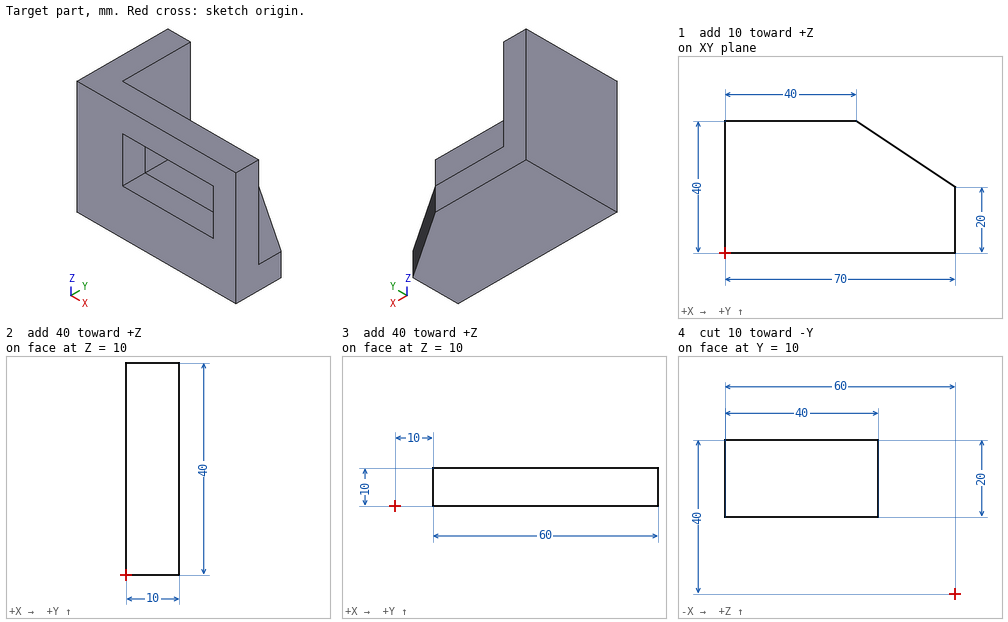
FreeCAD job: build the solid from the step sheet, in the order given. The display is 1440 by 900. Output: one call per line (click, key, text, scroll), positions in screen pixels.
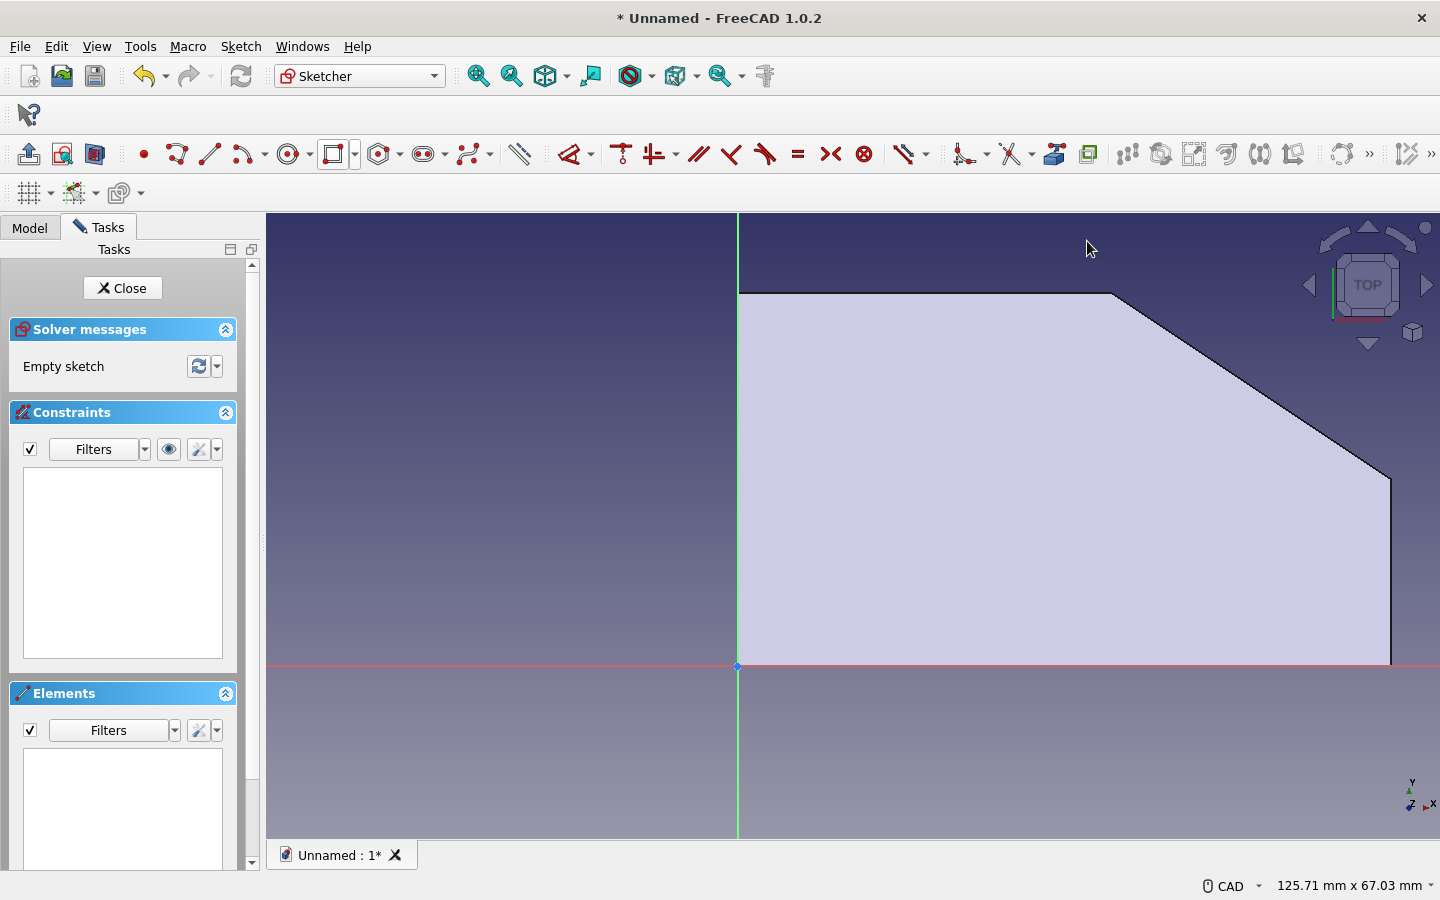
click(332, 154)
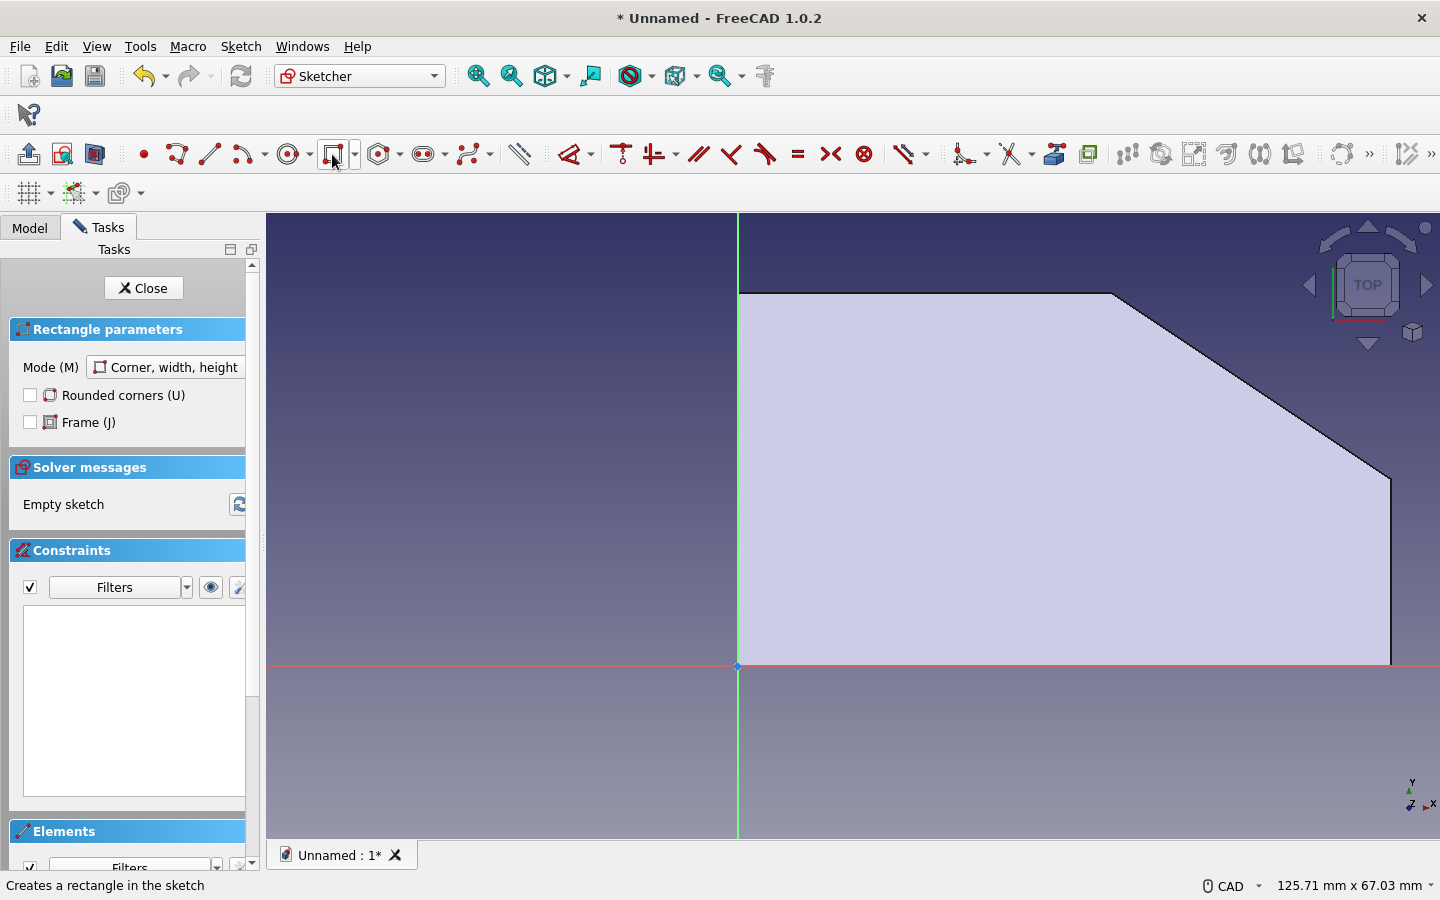
click(738, 666)
move(831, 293)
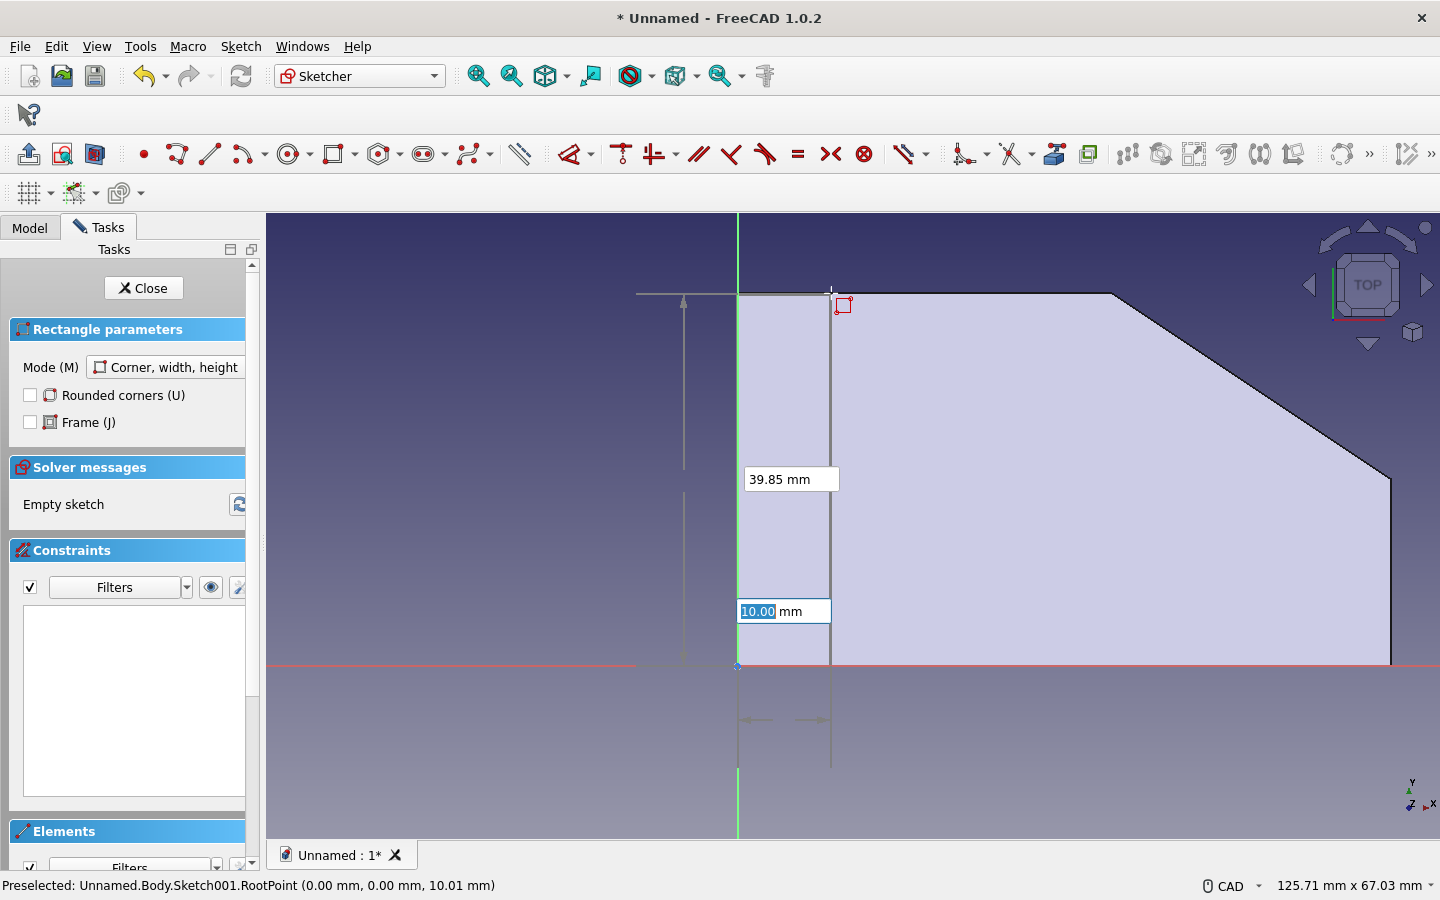
text(10)
key(Tab)
text(40)
key(Return)
key(Escape)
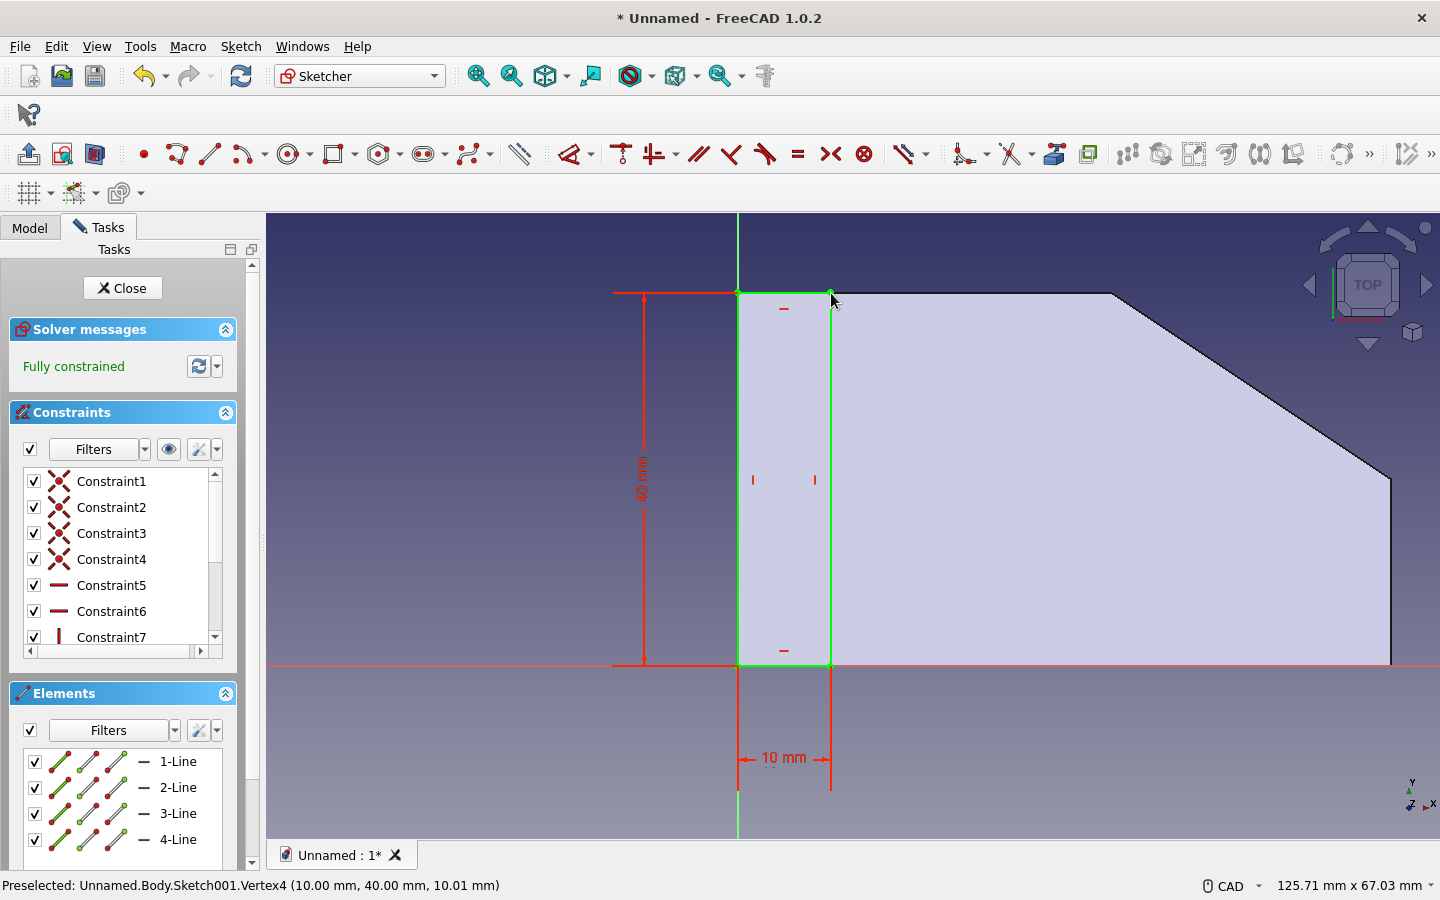
click(123, 288)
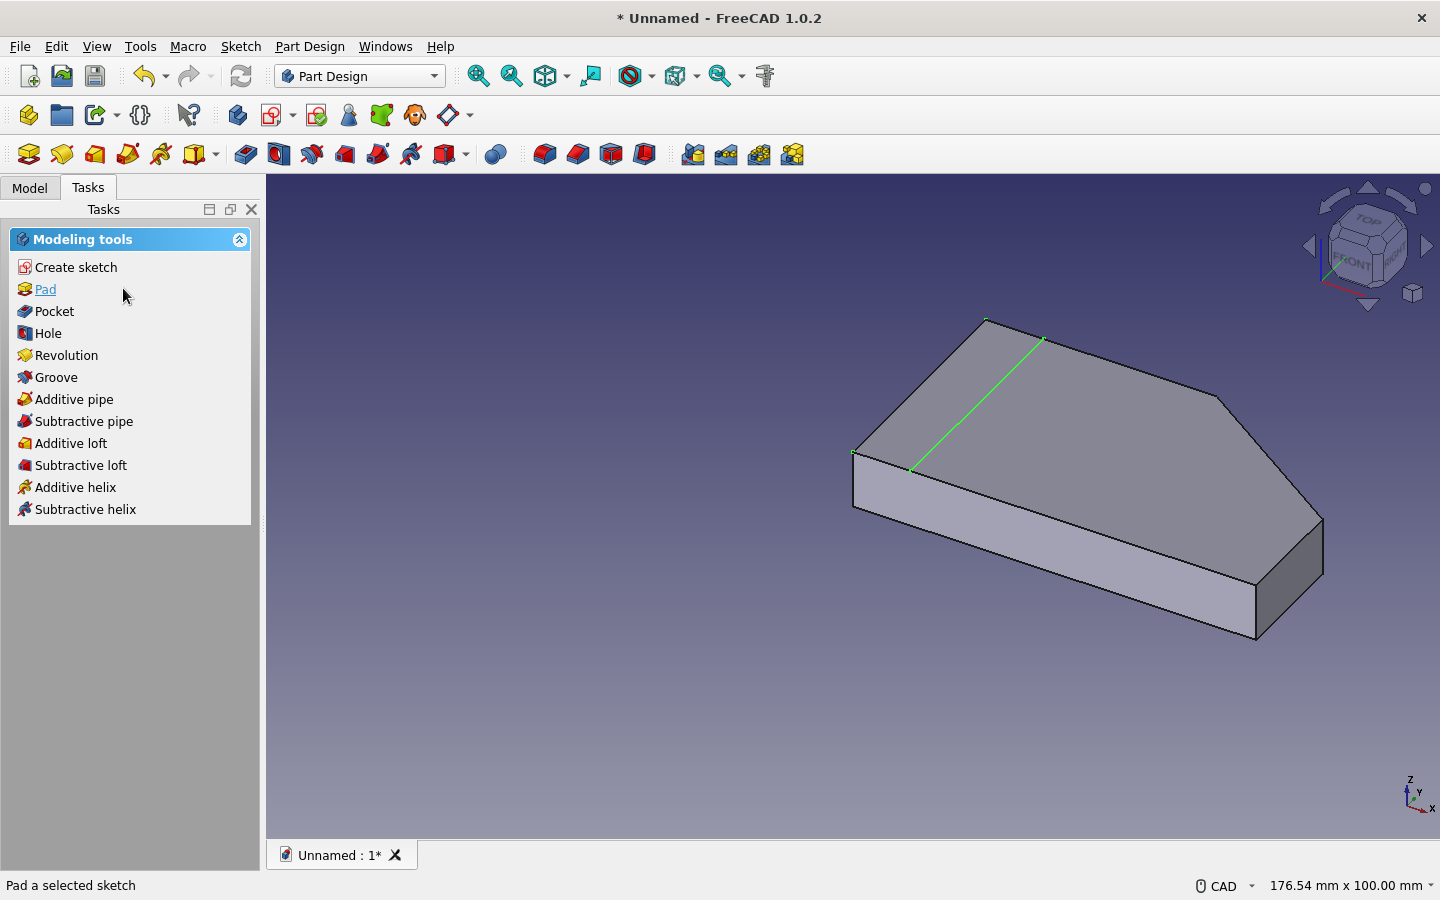
click(29, 154)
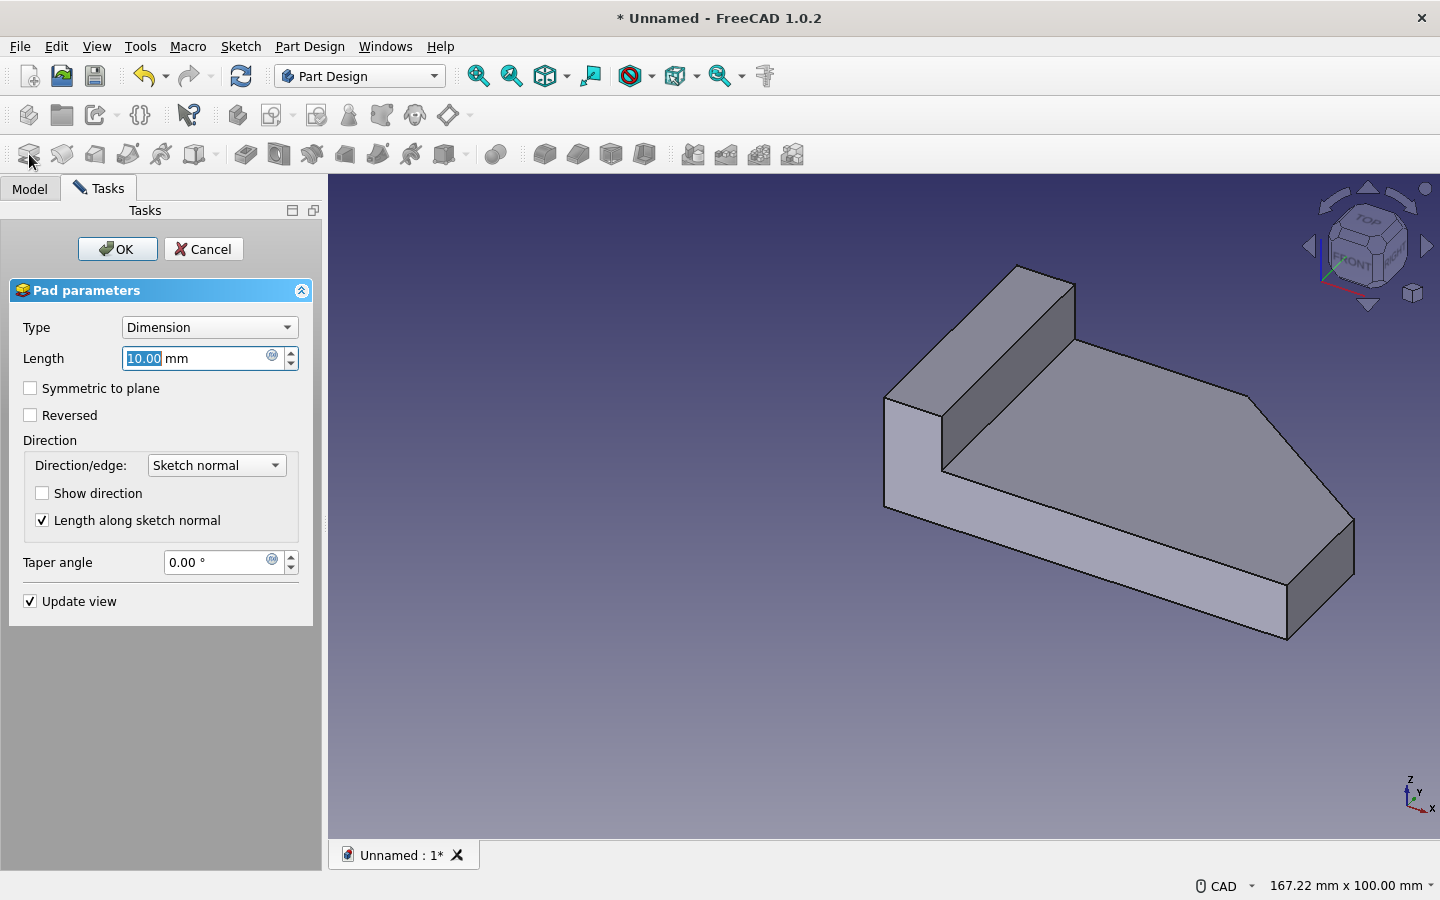
text(40)
key(Tab)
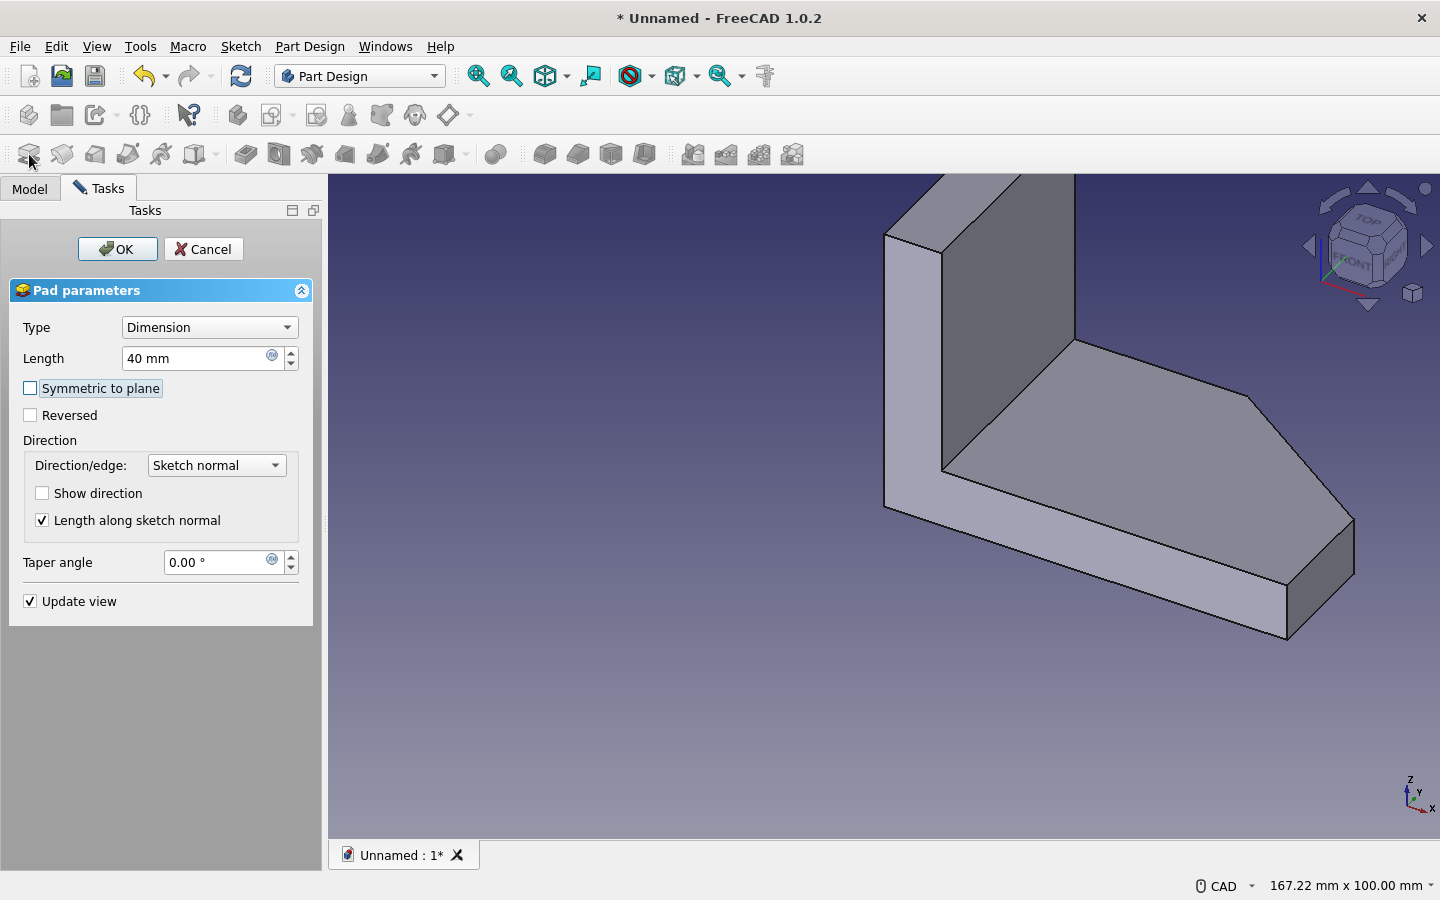
click(118, 249)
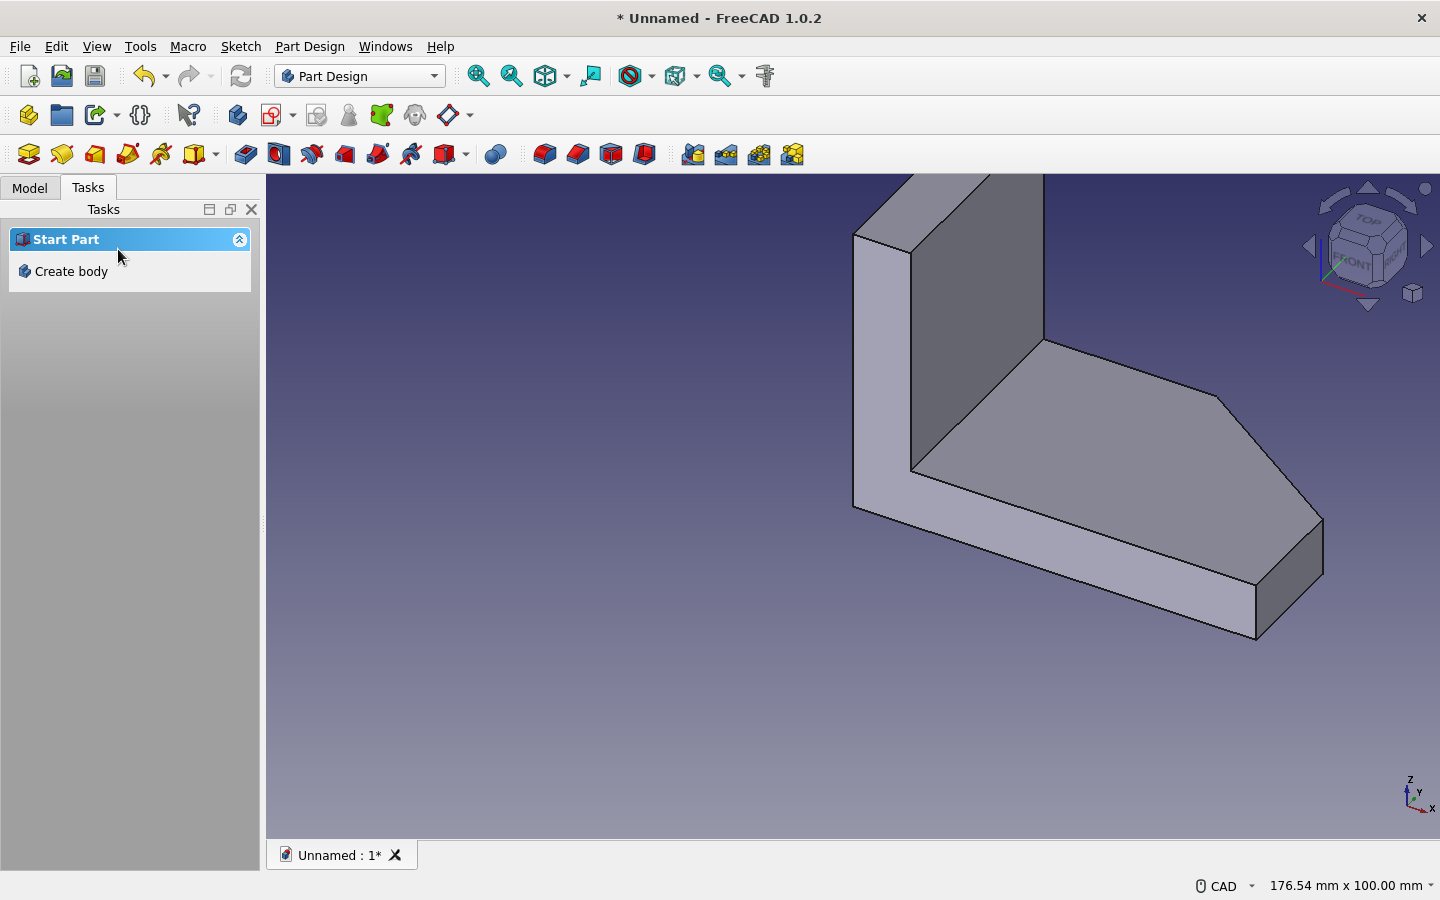
click(479, 76)